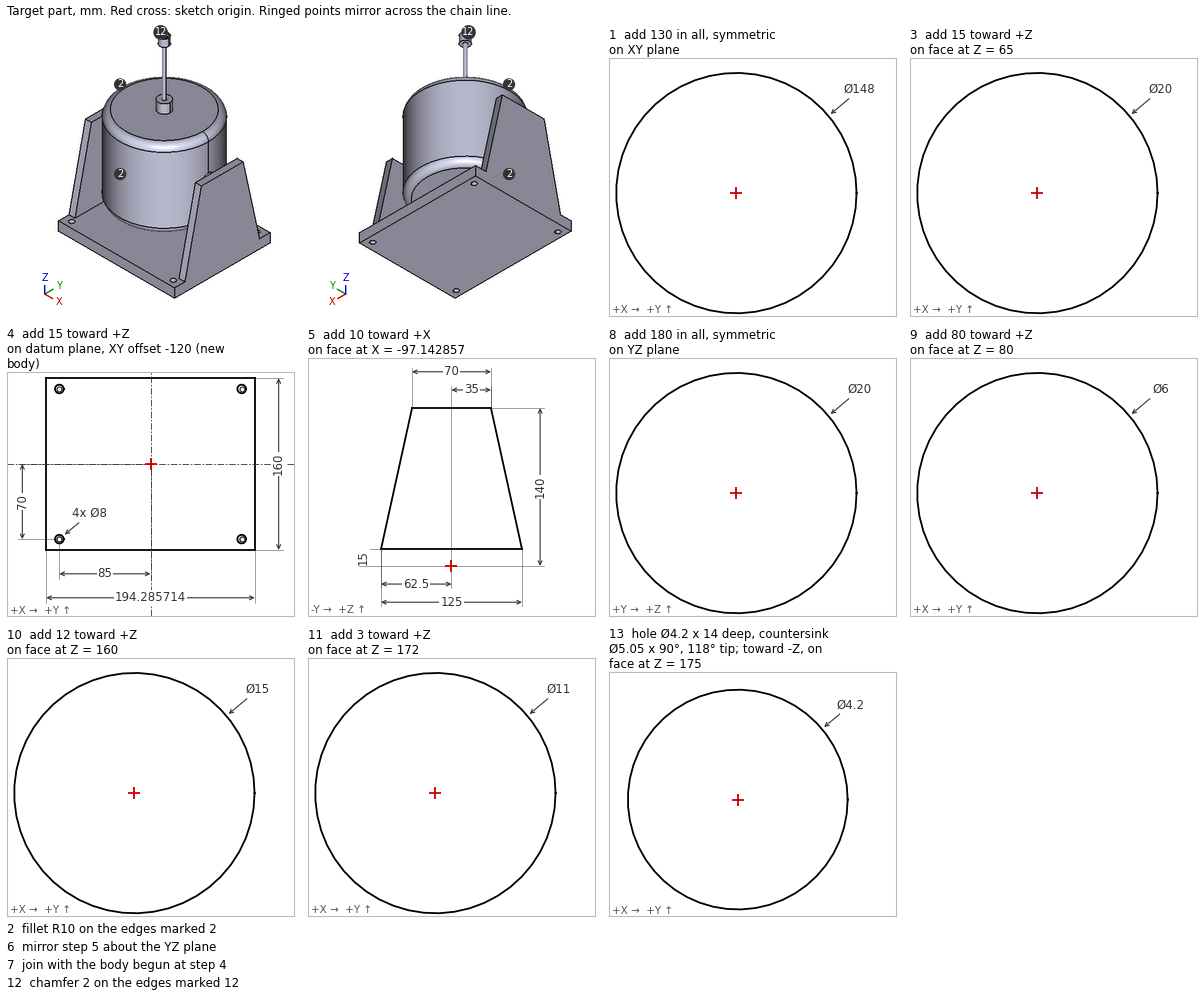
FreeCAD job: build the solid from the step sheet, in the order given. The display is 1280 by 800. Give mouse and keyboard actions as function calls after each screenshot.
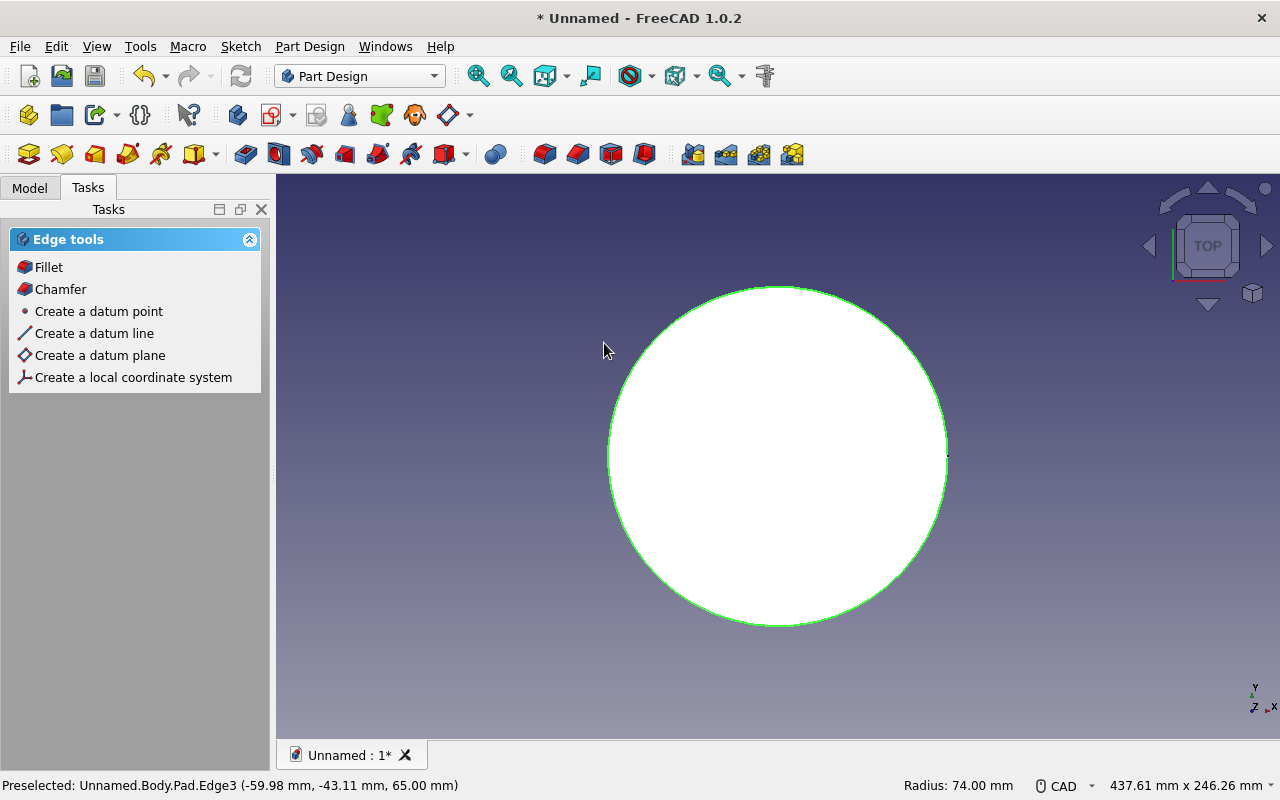
key(1)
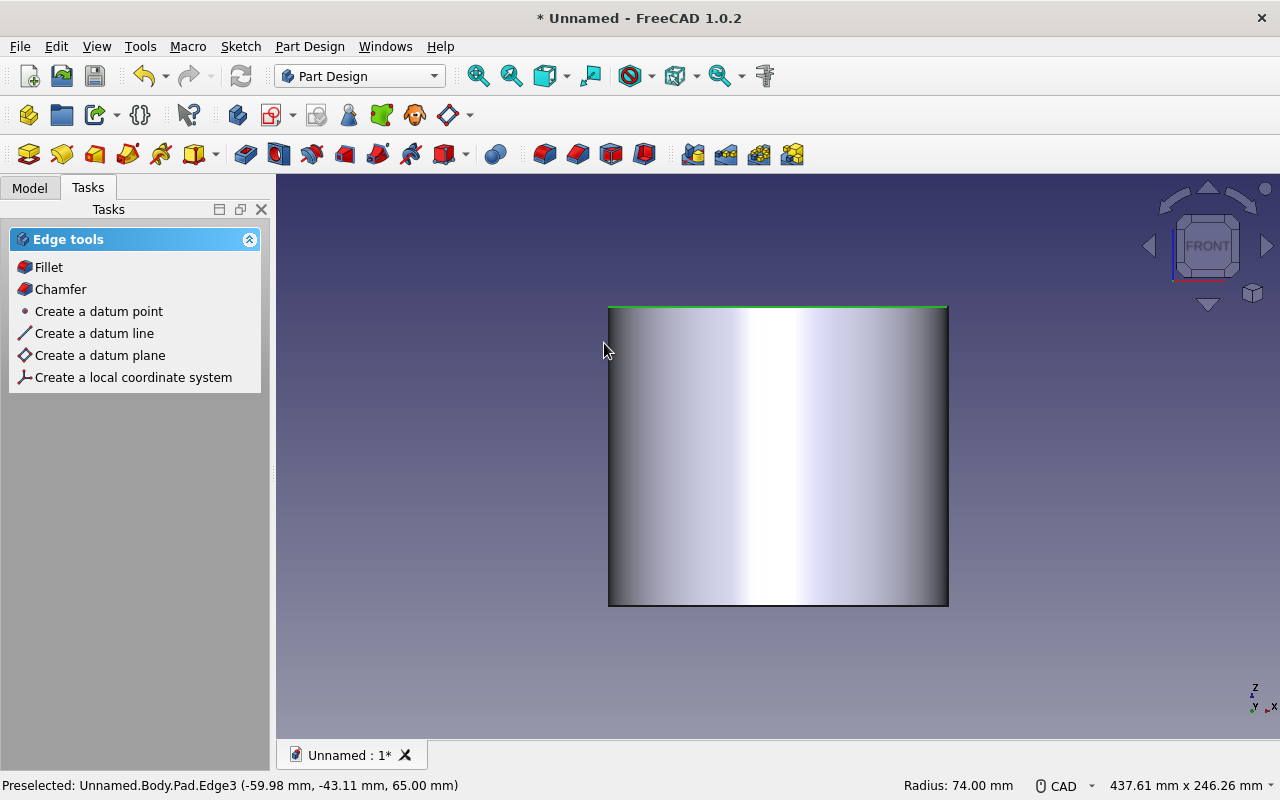
click(640, 605, ctrl)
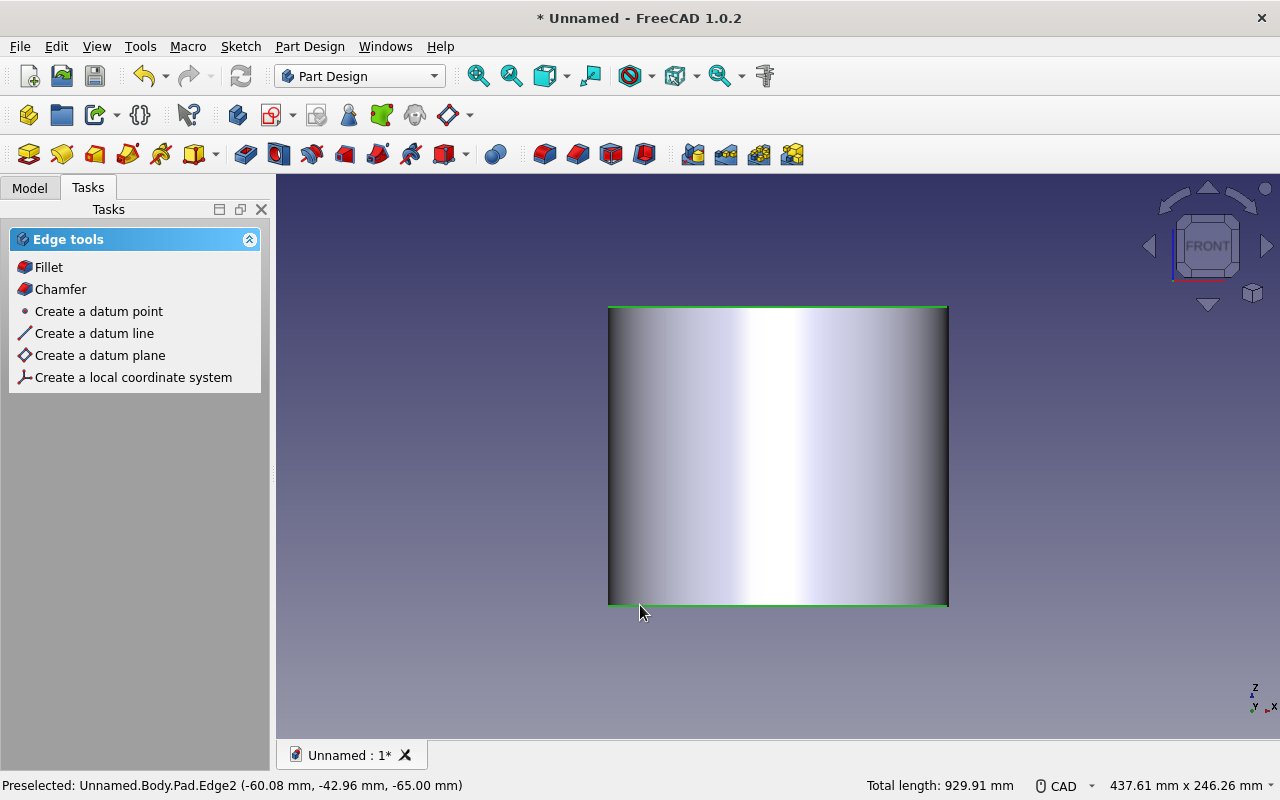
click(545, 154)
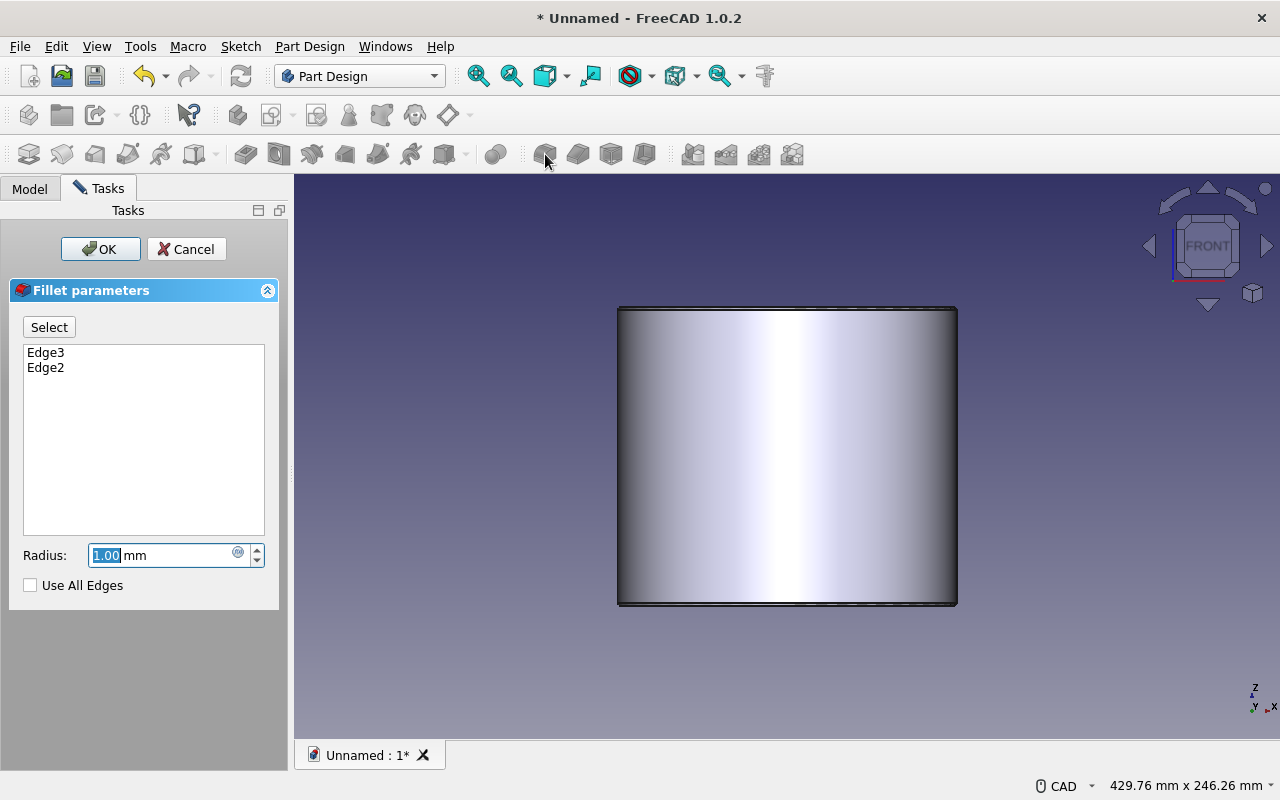
text(10)
key(Tab)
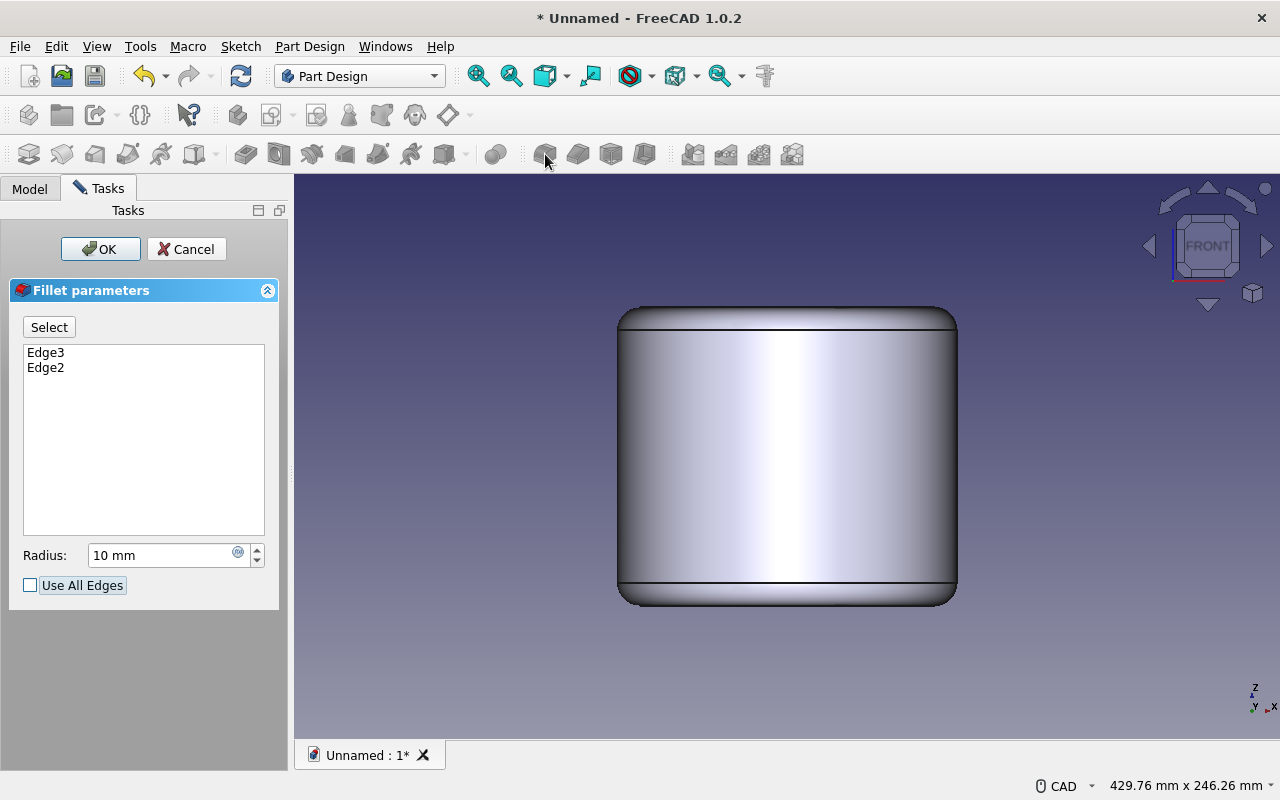
click(101, 249)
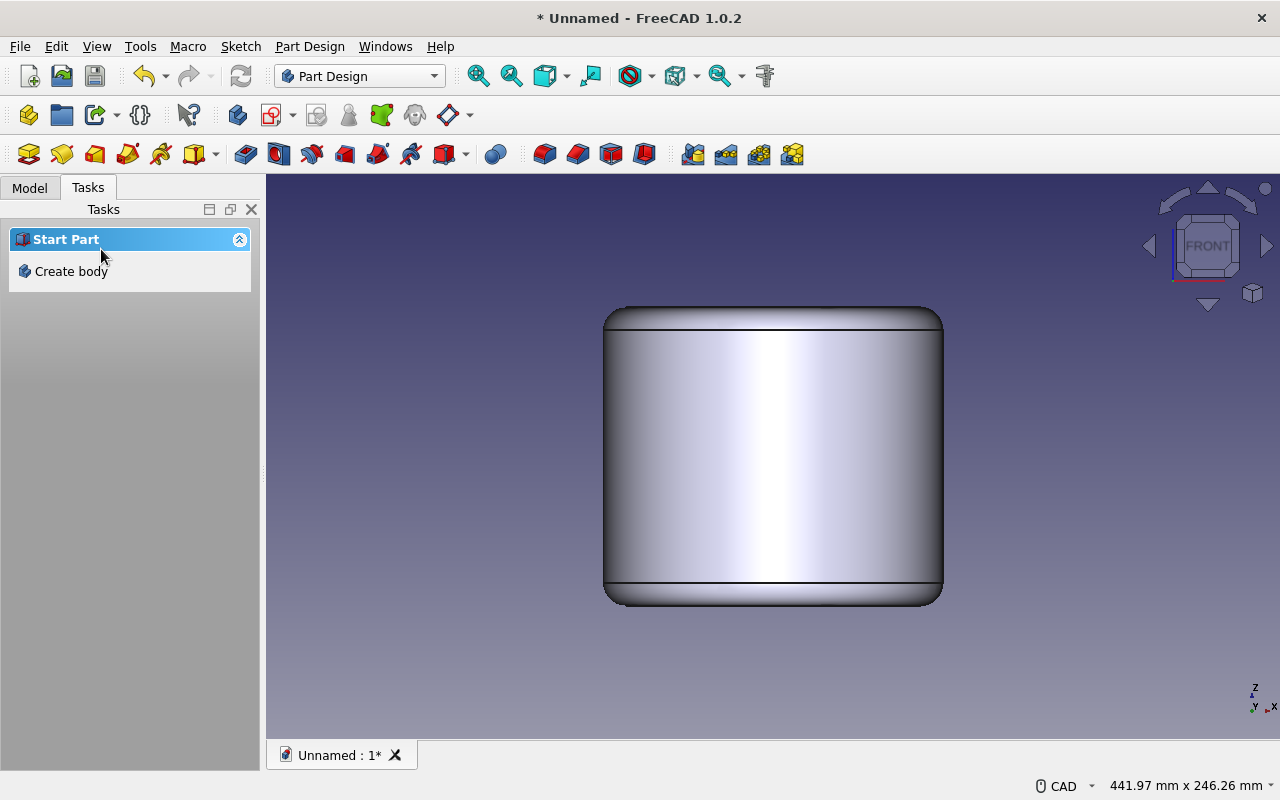
key(0)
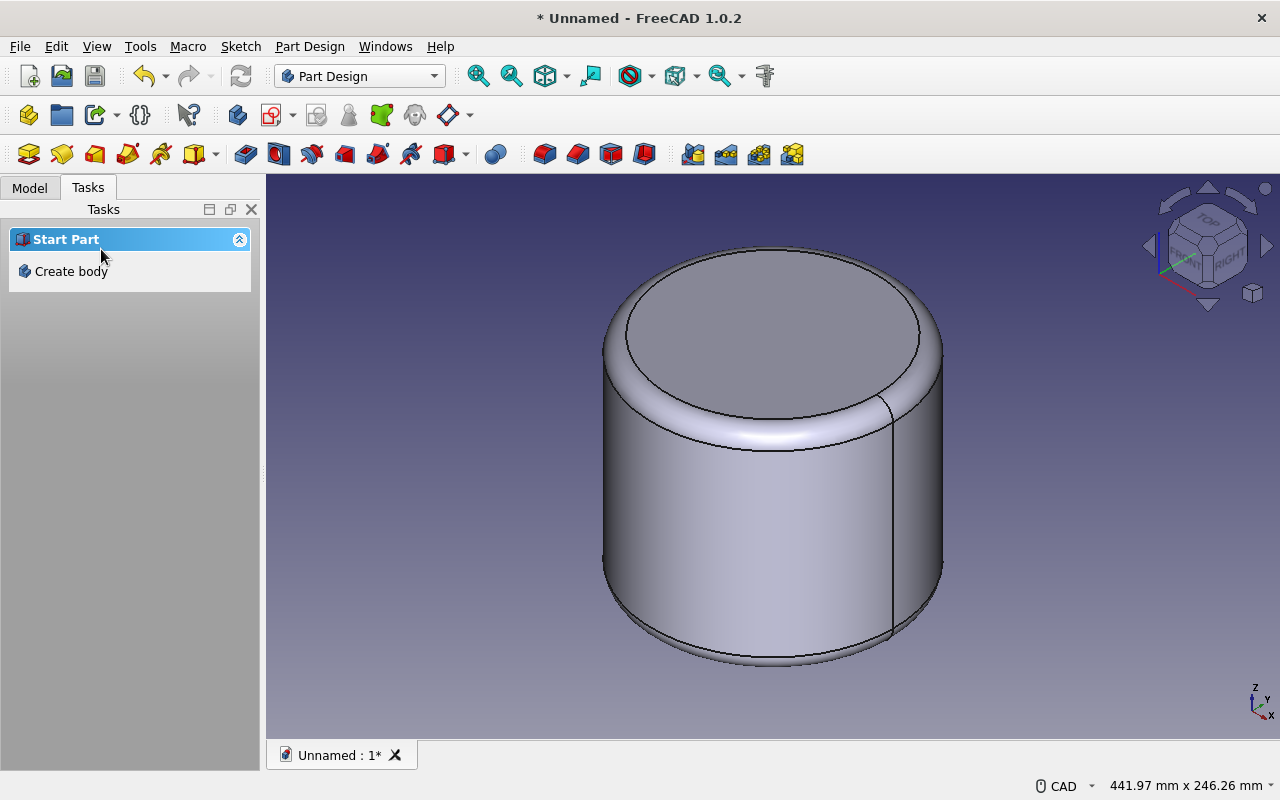
click(773, 334)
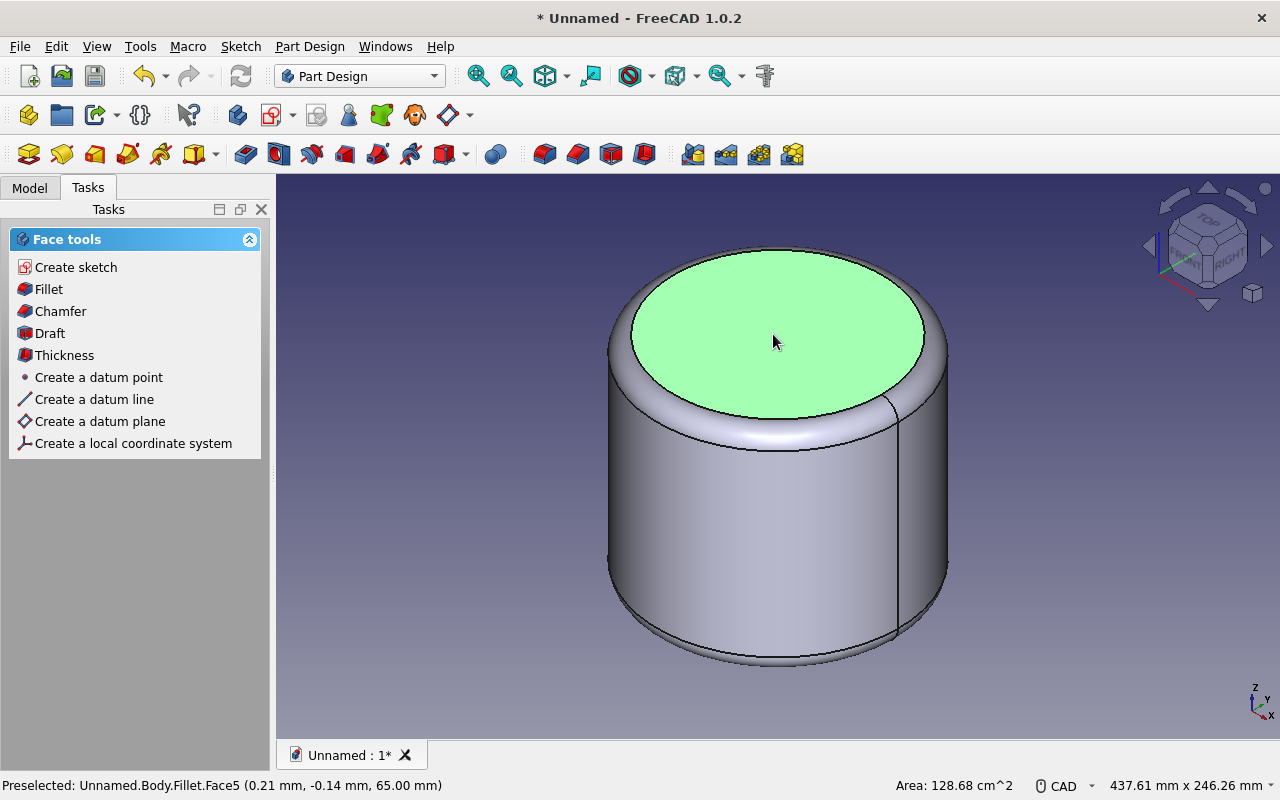
click(270, 116)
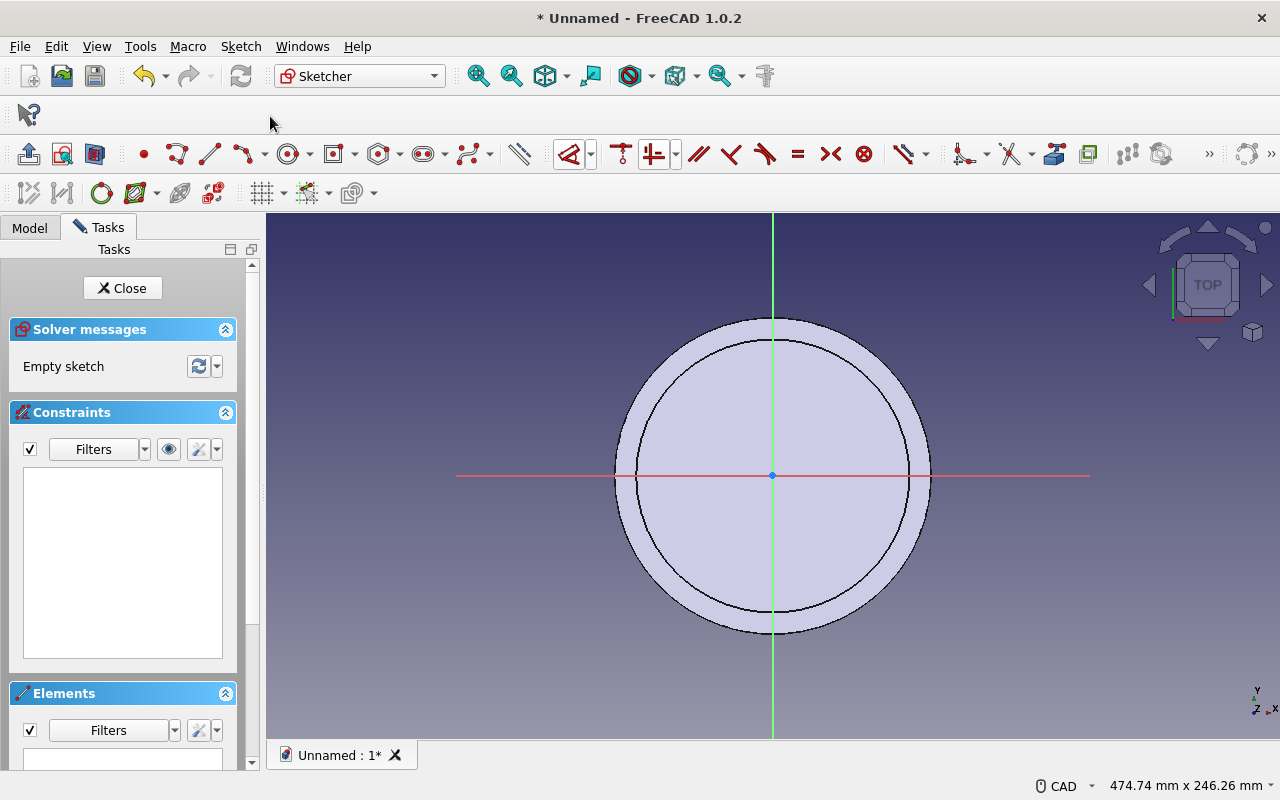
scroll(784, 476, up, 10)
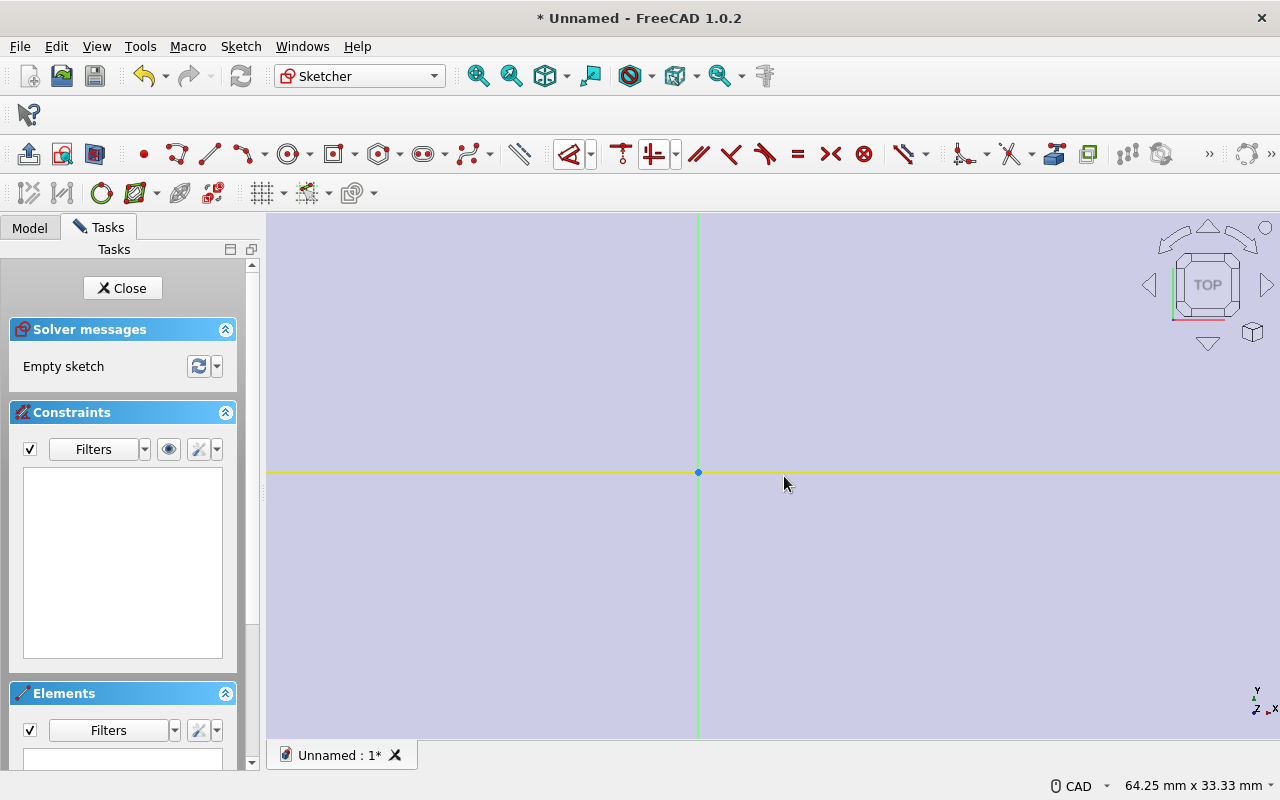
click(288, 154)